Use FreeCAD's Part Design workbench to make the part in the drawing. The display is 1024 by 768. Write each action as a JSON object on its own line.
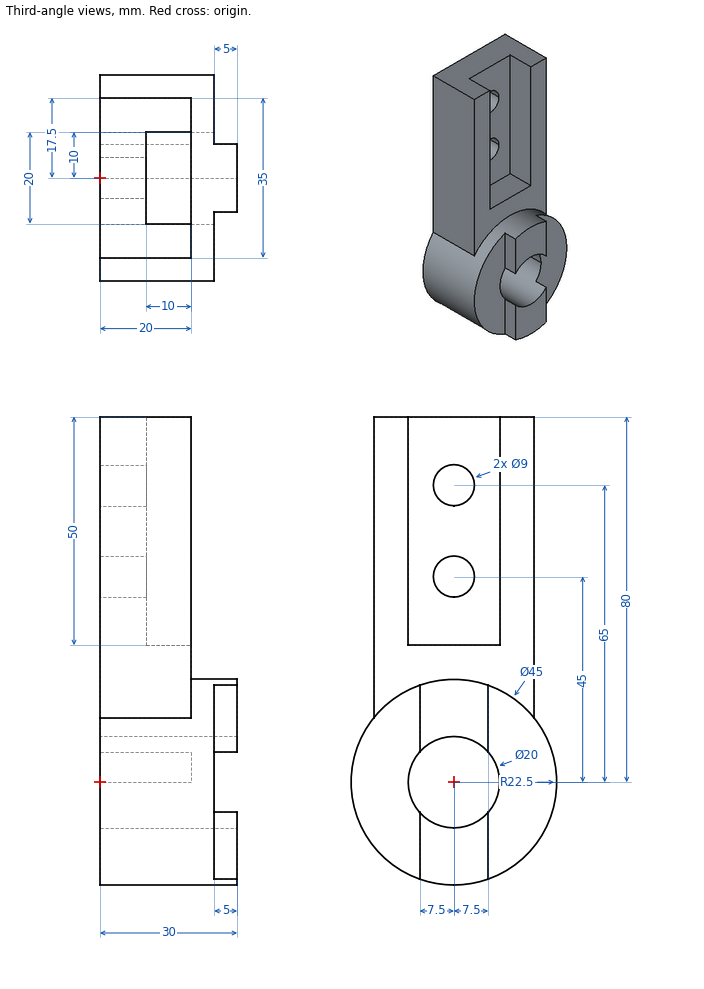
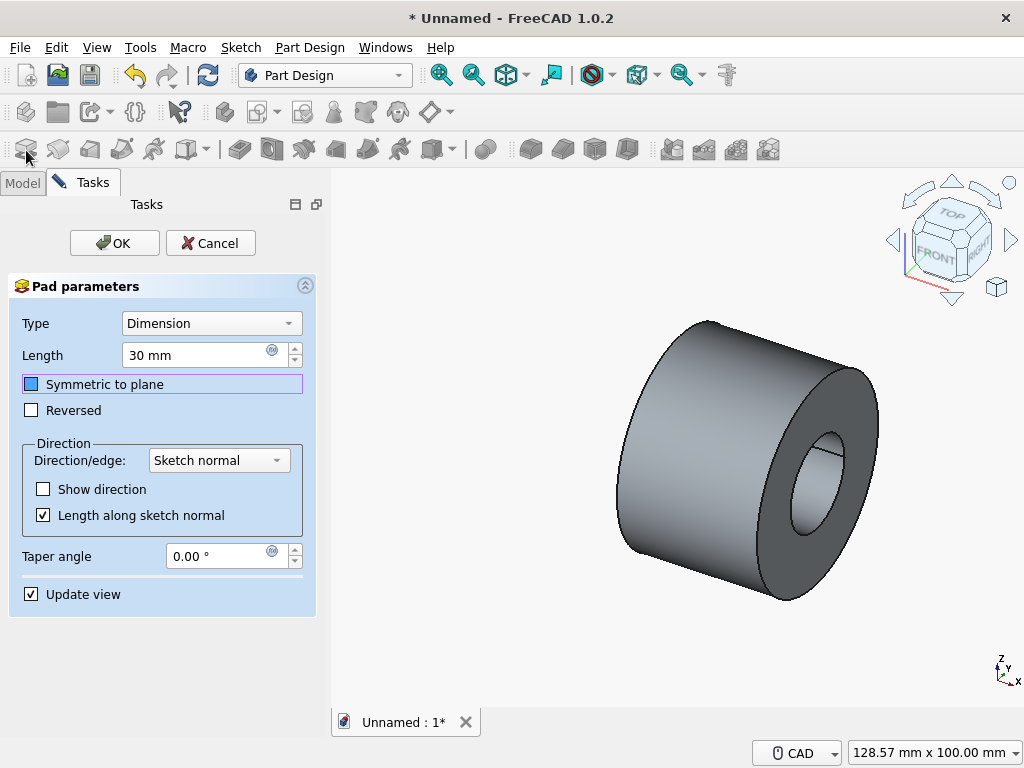
{"action": "left_click", "coordinate": [115, 243]}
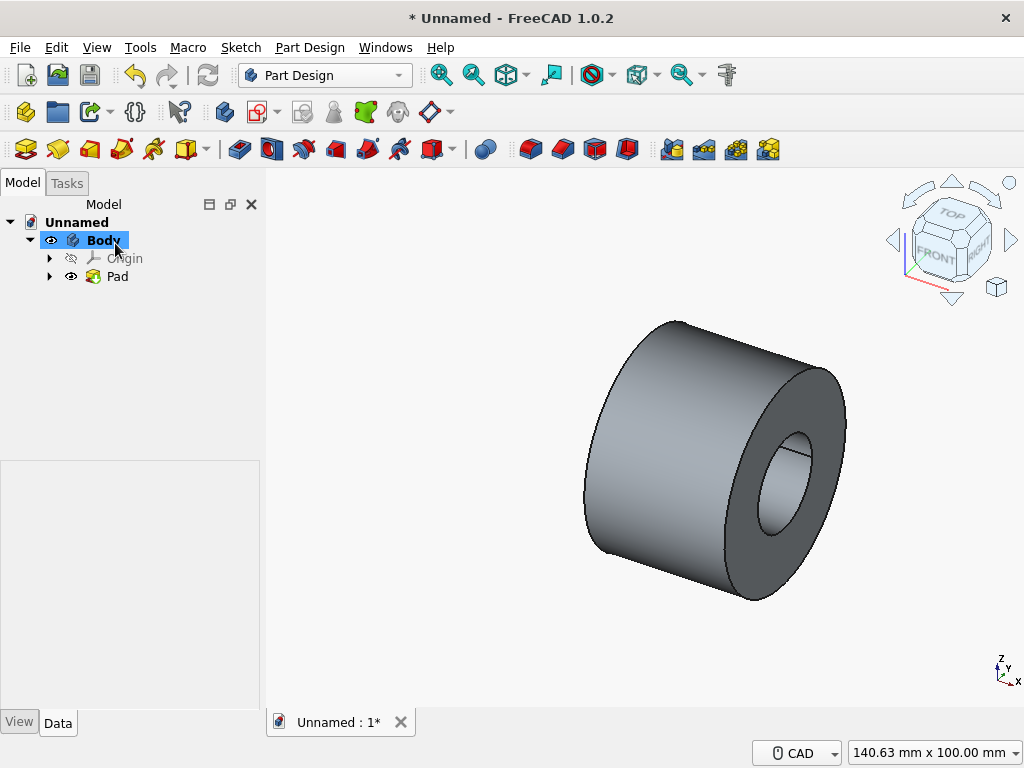
{"action": "left_click", "coordinate": [50, 258]}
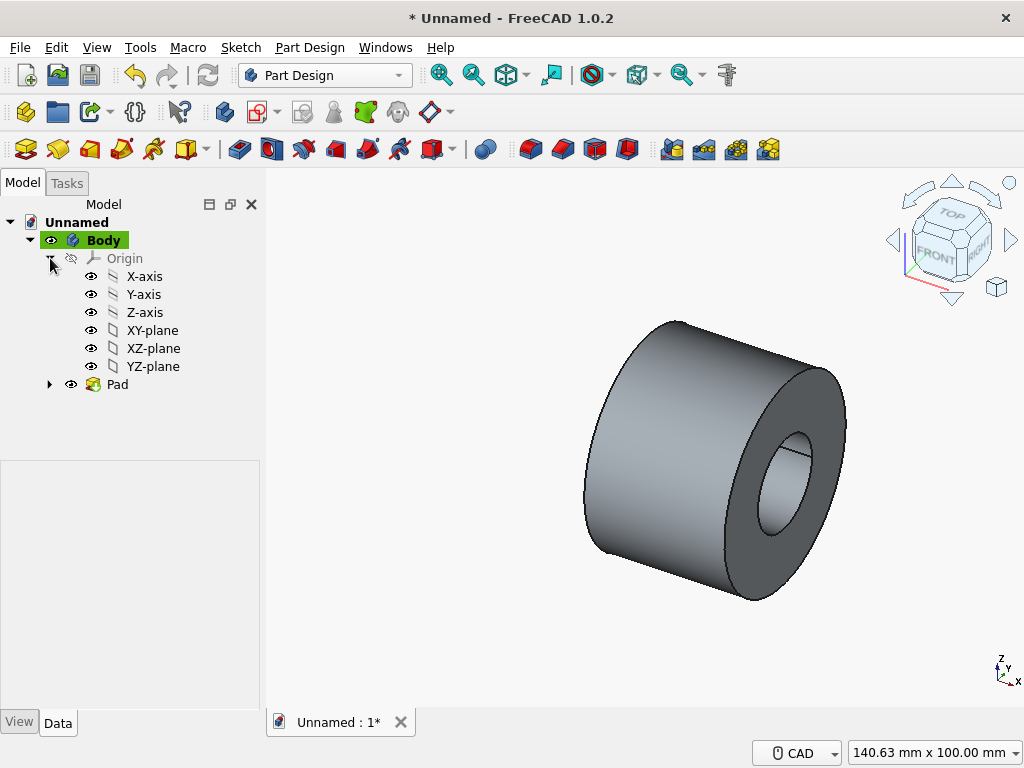
{"action": "left_click", "coordinate": [136, 366]}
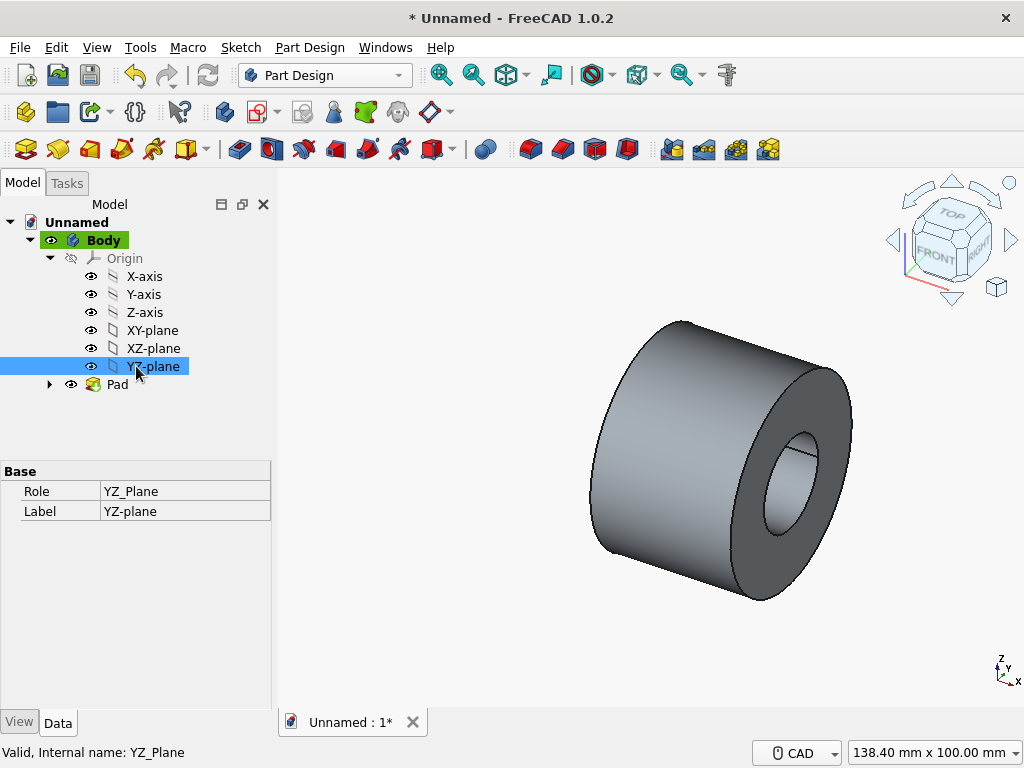
{"action": "left_click", "coordinate": [430, 112]}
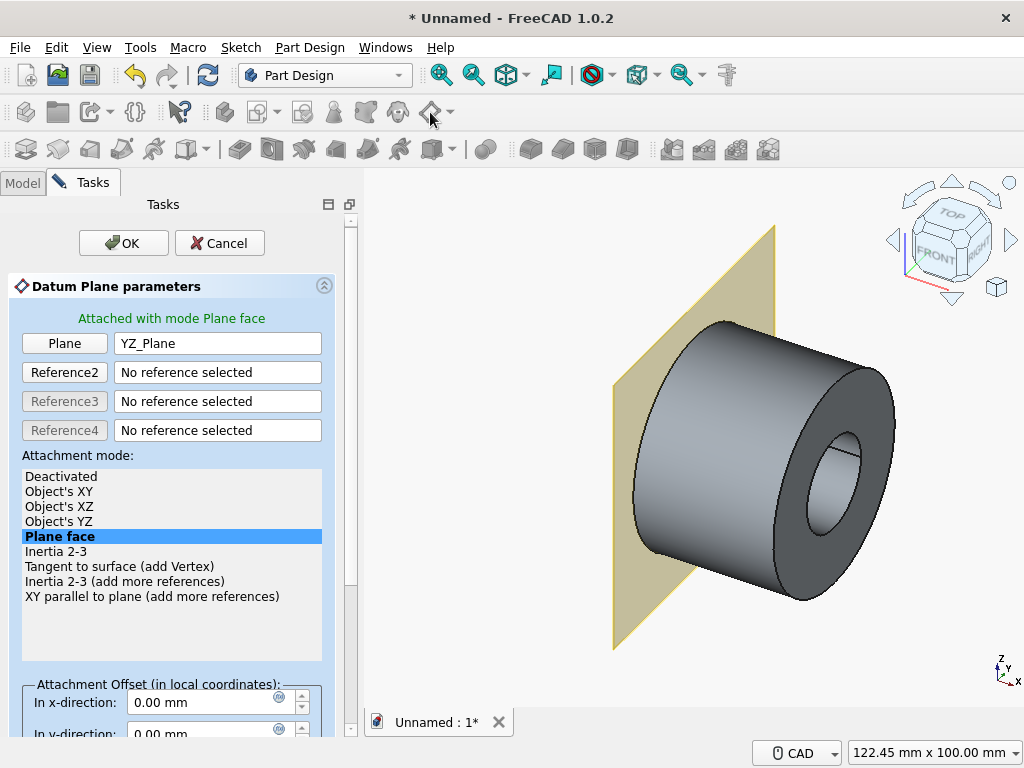
{"action": "scroll", "coordinate": [351, 475], "scroll_direction": "down", "scroll_amount": 2}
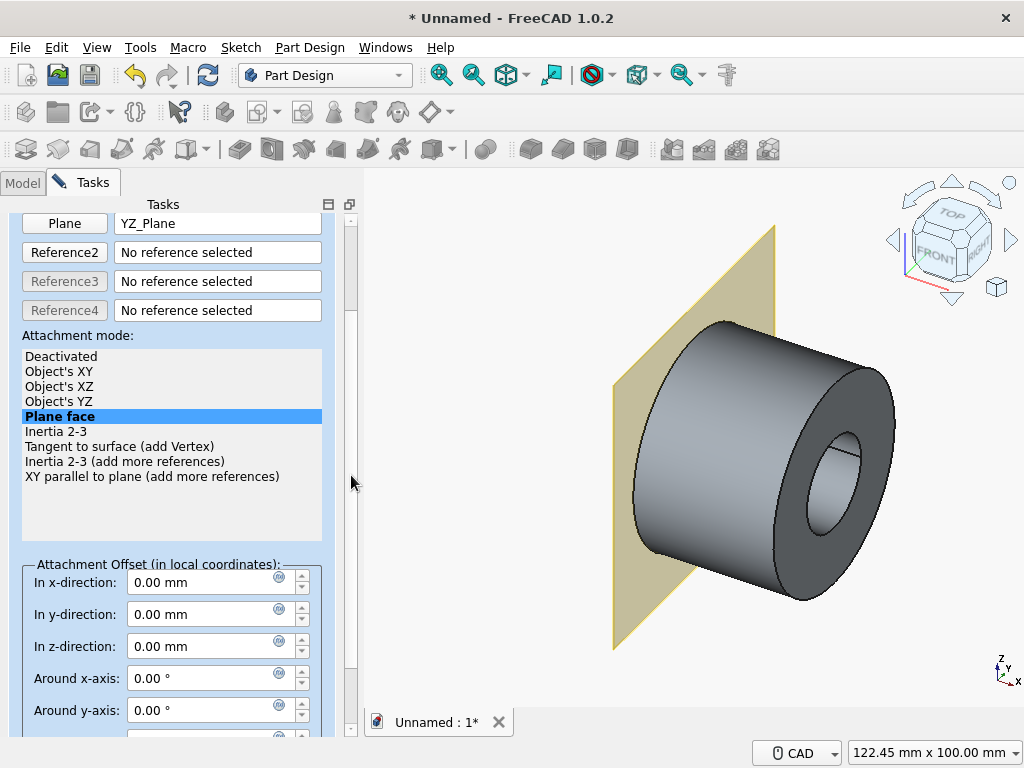
{"action": "triple_click", "coordinate": [210, 646]}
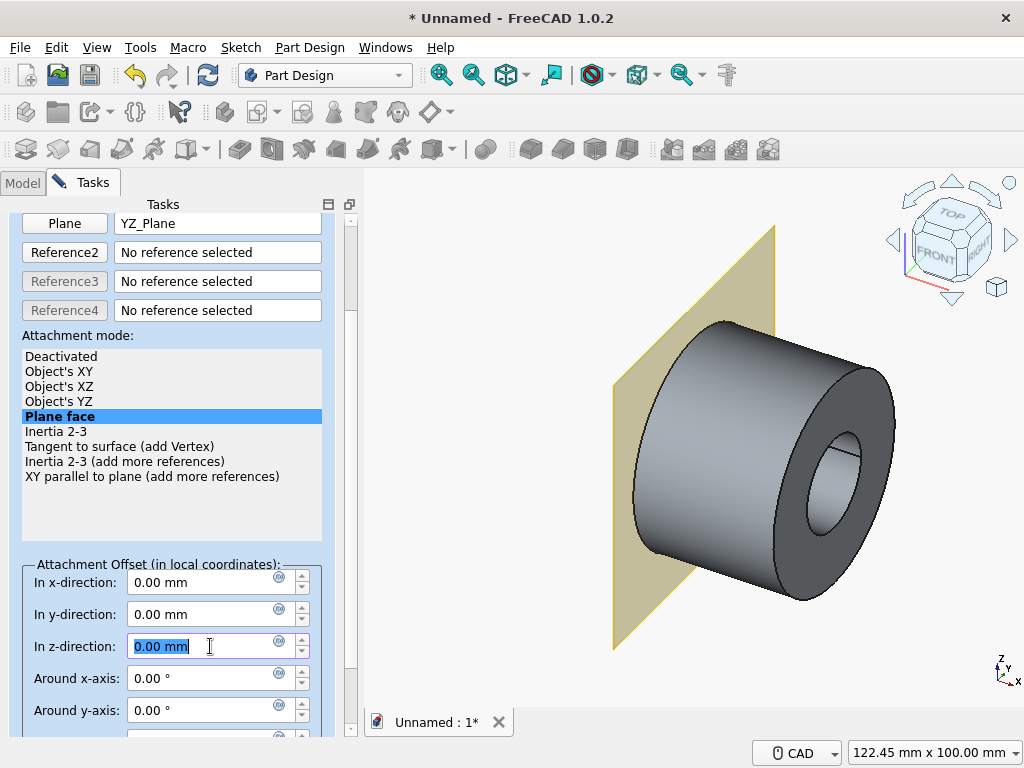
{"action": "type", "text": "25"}
{"action": "key", "text": "Tab"}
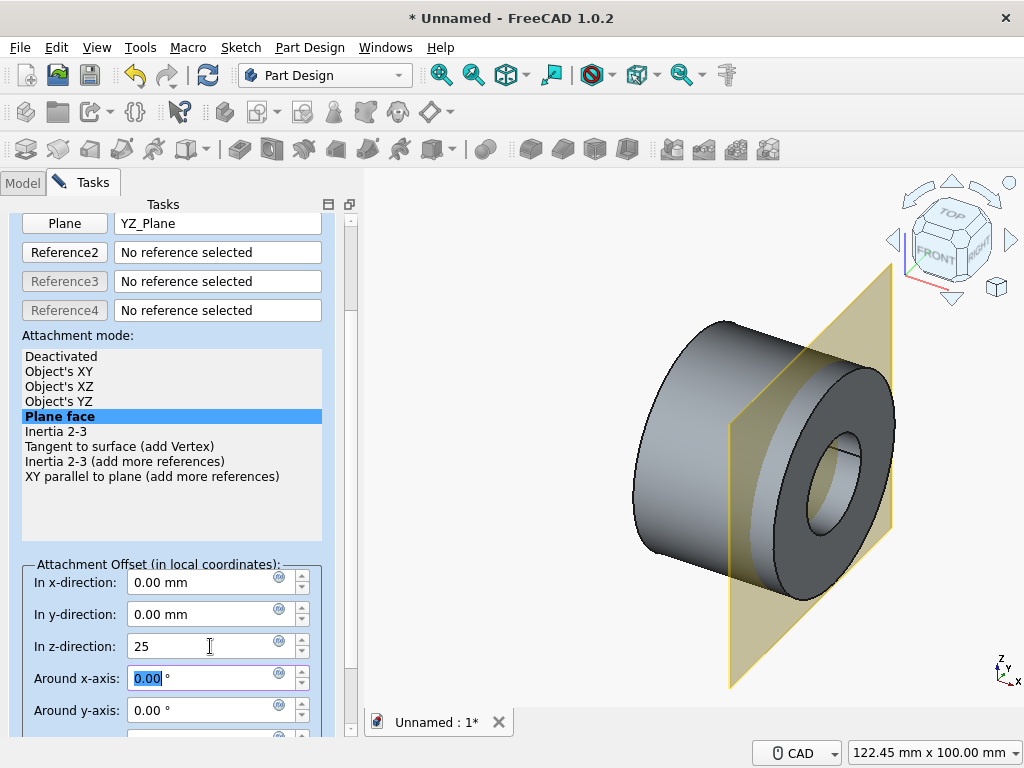
{"action": "scroll", "coordinate": [351, 475], "scroll_direction": "up", "scroll_amount": 3}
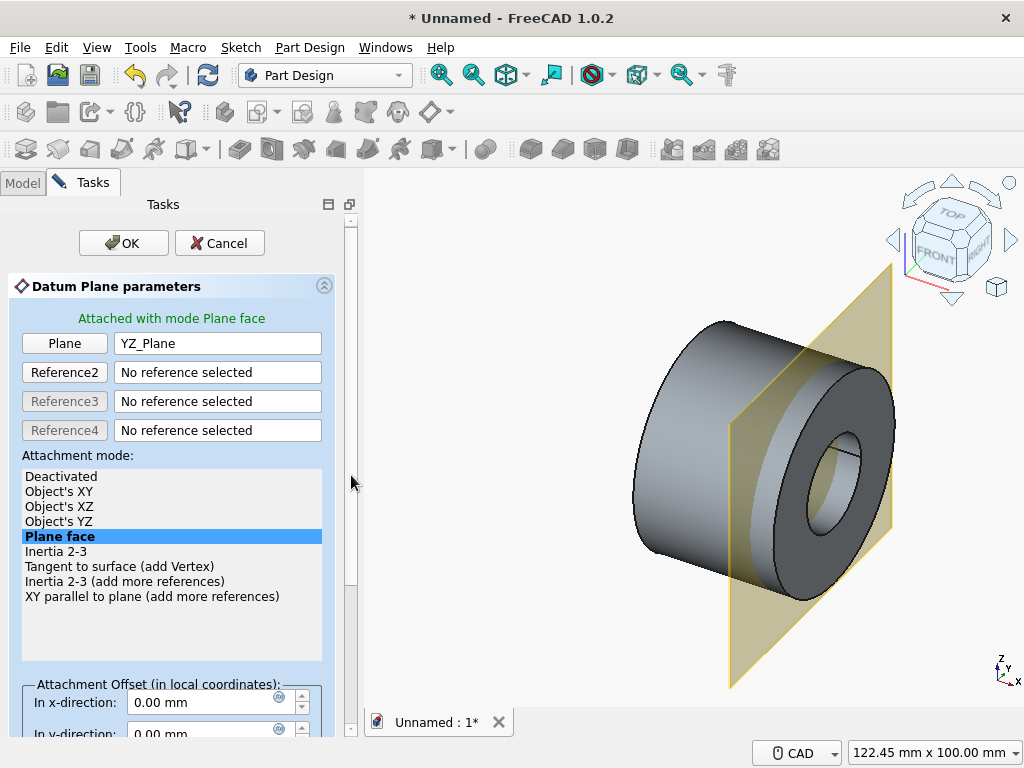
{"action": "left_click", "coordinate": [124, 243]}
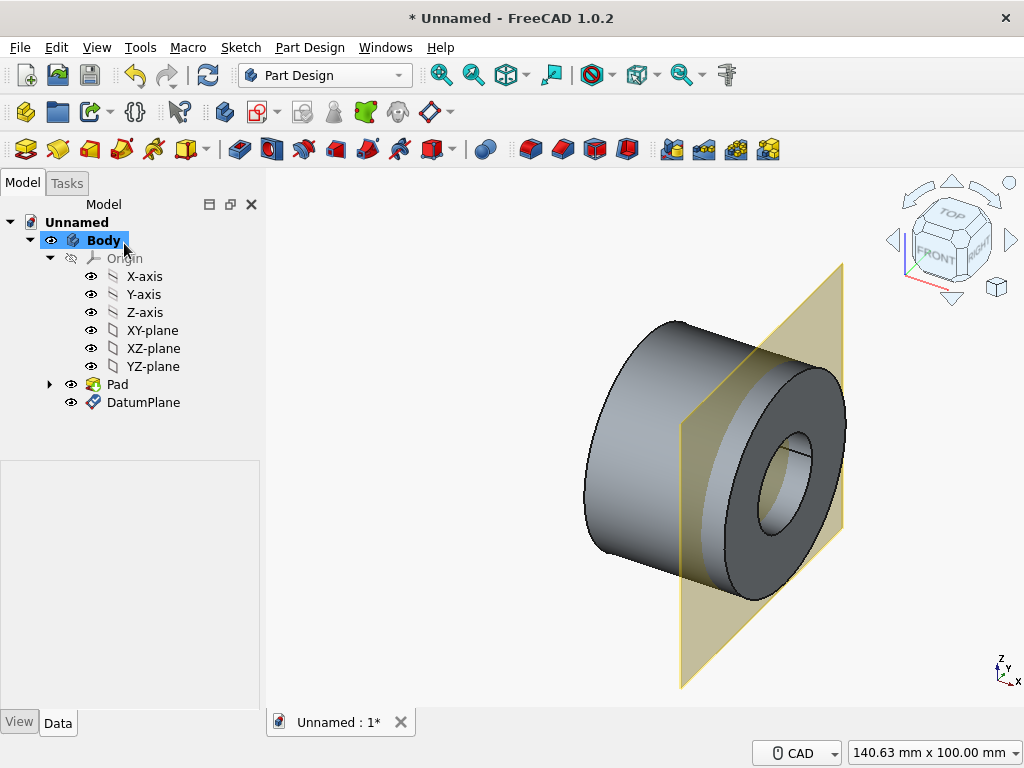
{"action": "left_click", "coordinate": [116, 402]}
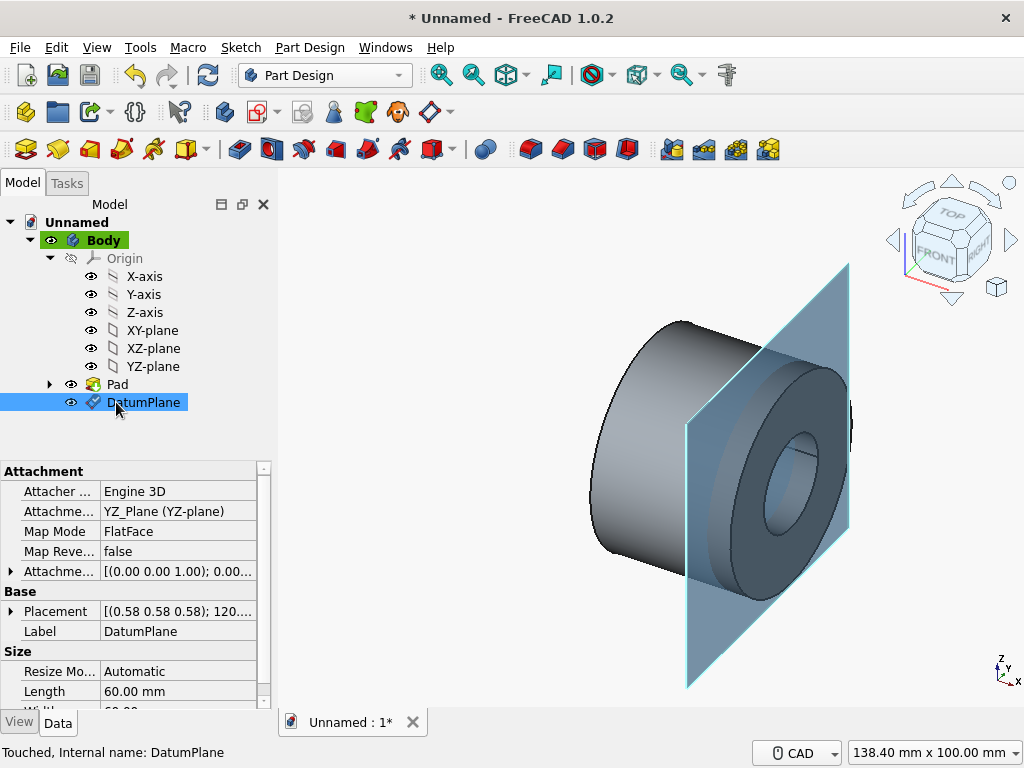
{"action": "left_click", "coordinate": [258, 112]}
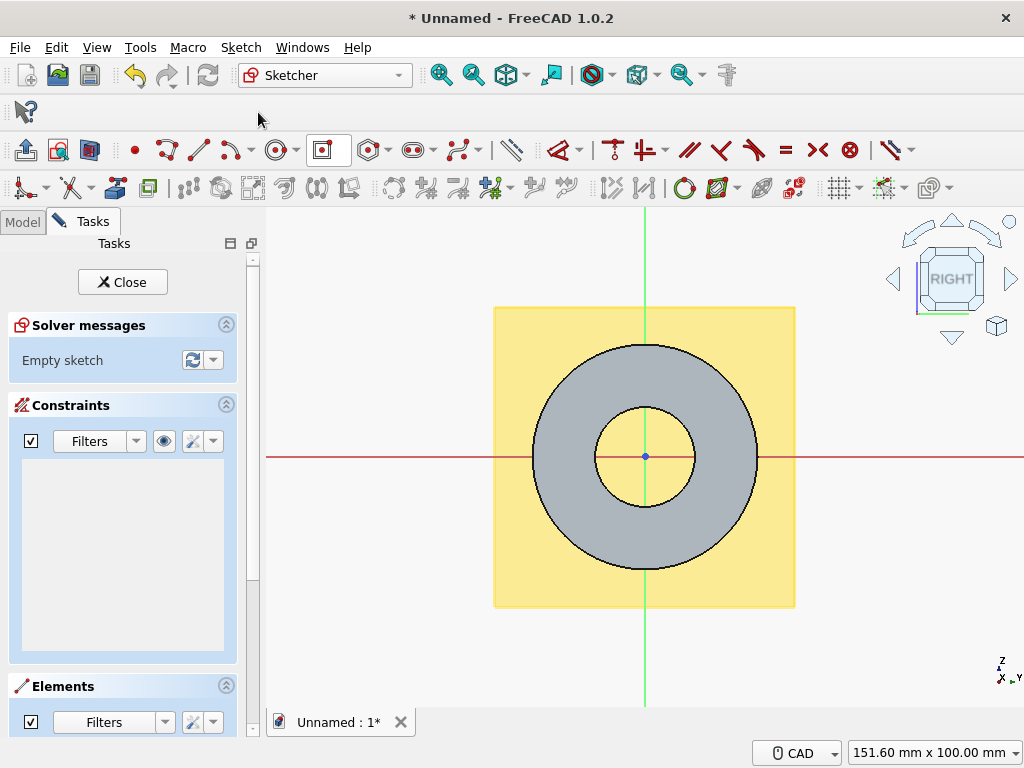
{"action": "left_click", "coordinate": [90, 150]}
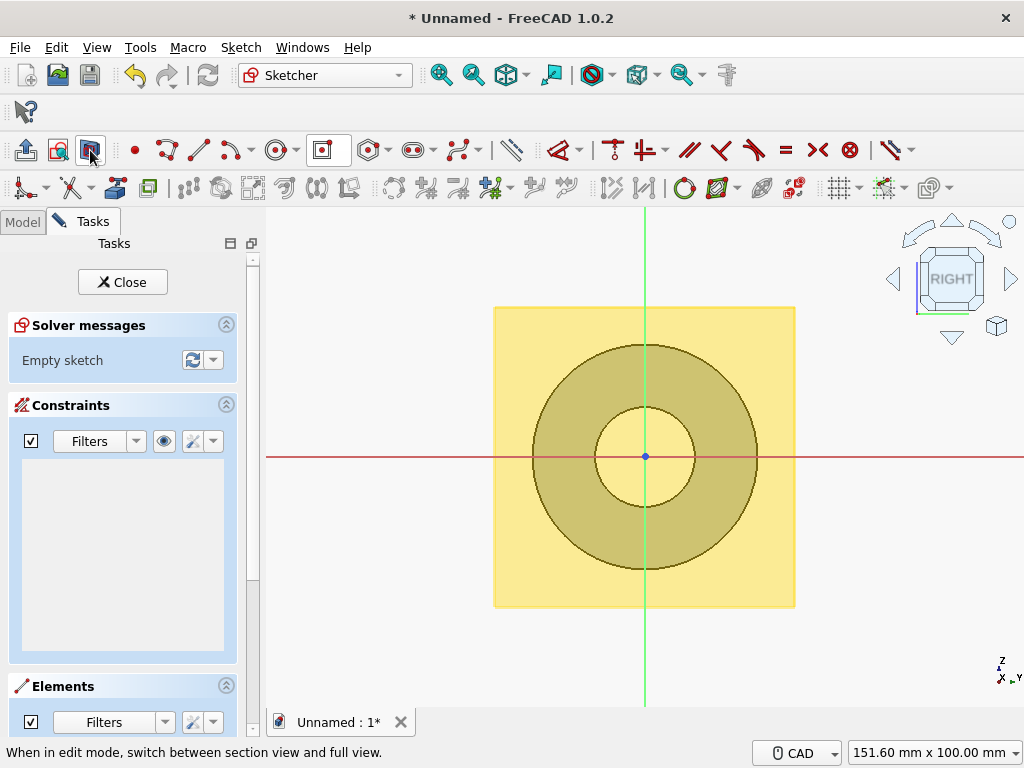
{"action": "scroll", "coordinate": [859, 457], "scroll_direction": "up", "scroll_amount": 2}